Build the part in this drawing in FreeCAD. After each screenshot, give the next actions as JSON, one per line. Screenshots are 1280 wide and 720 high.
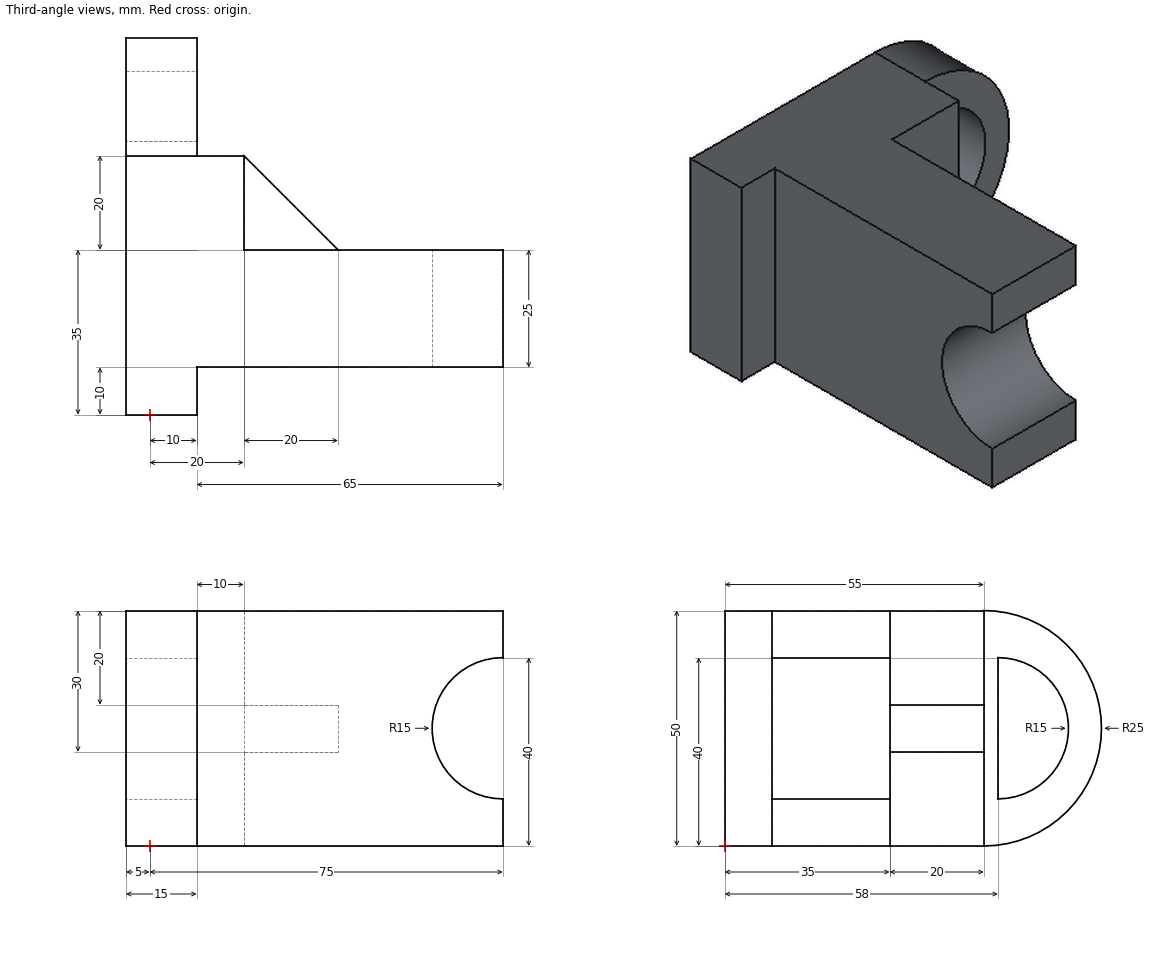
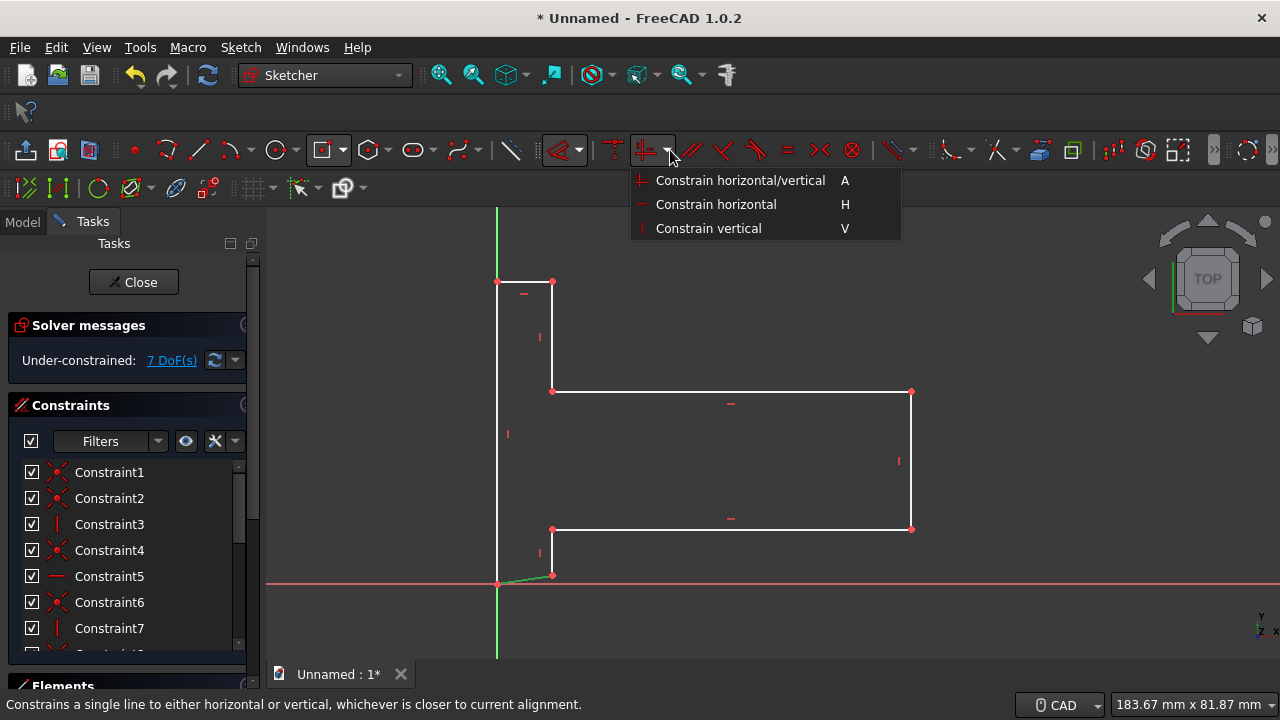
{"action": "left_click", "coordinate": [766, 204]}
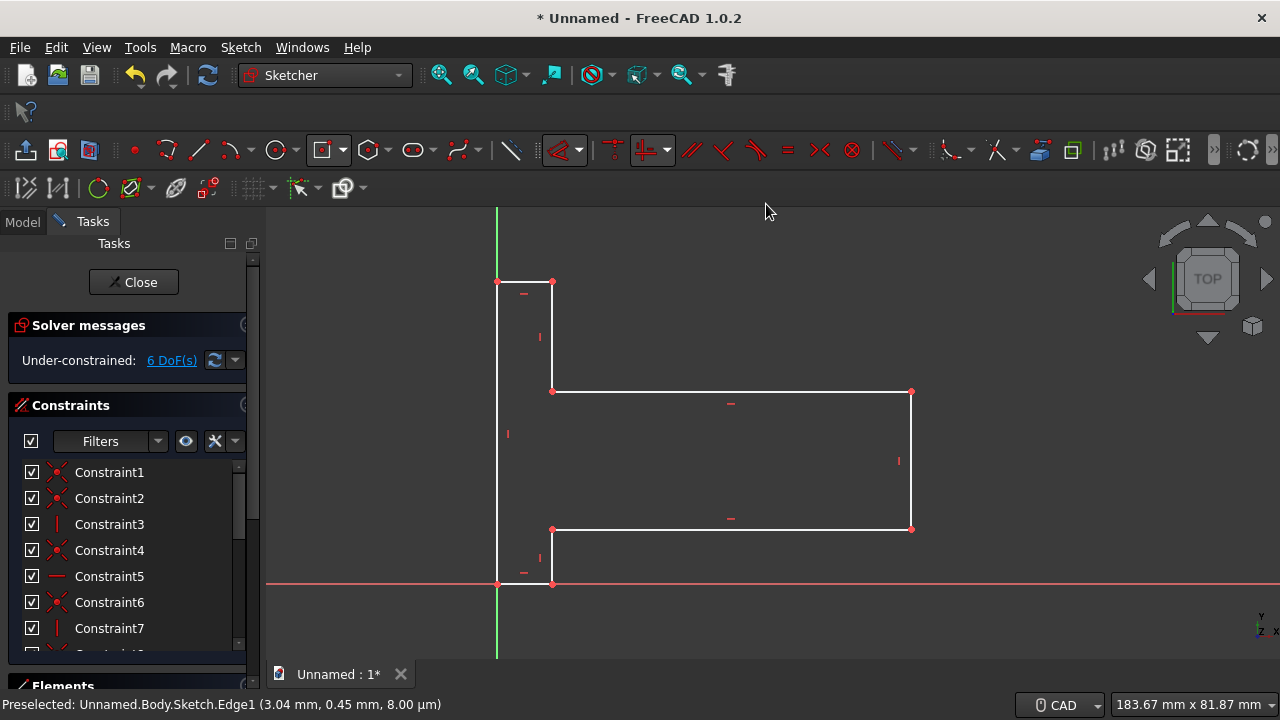
{"action": "left_click", "coordinate": [514, 584]}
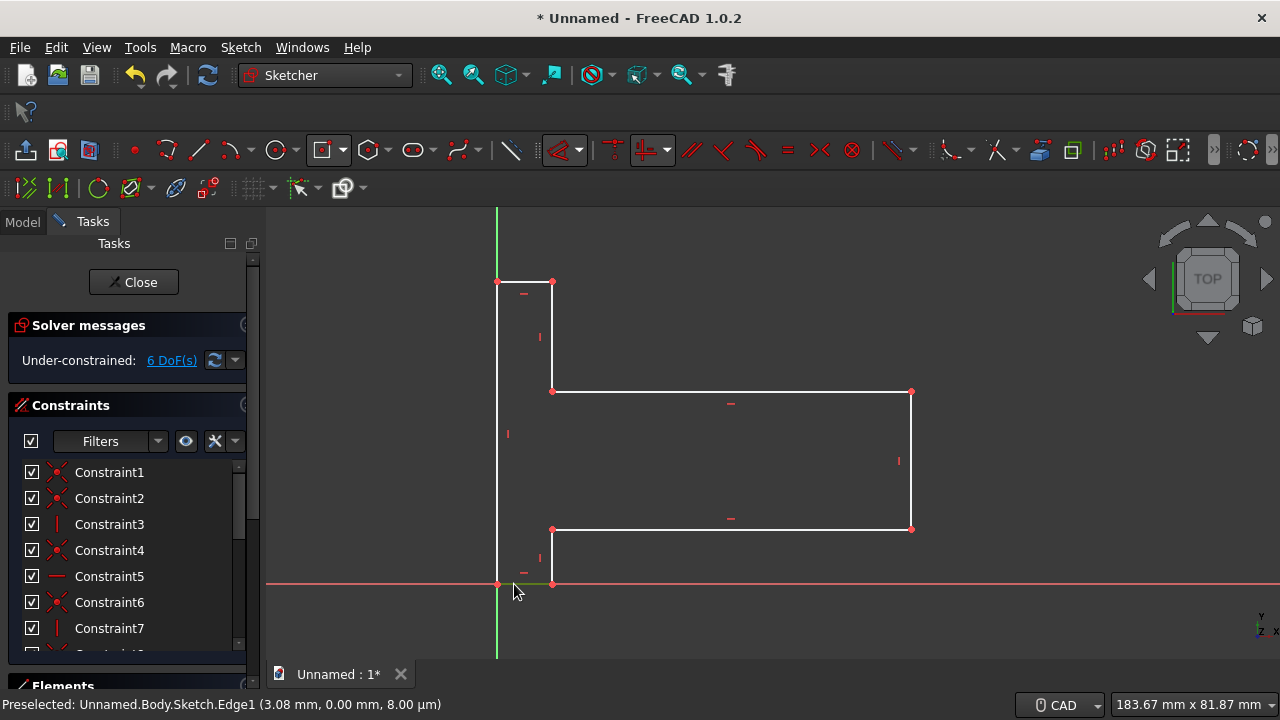
{"action": "left_click", "coordinate": [582, 150]}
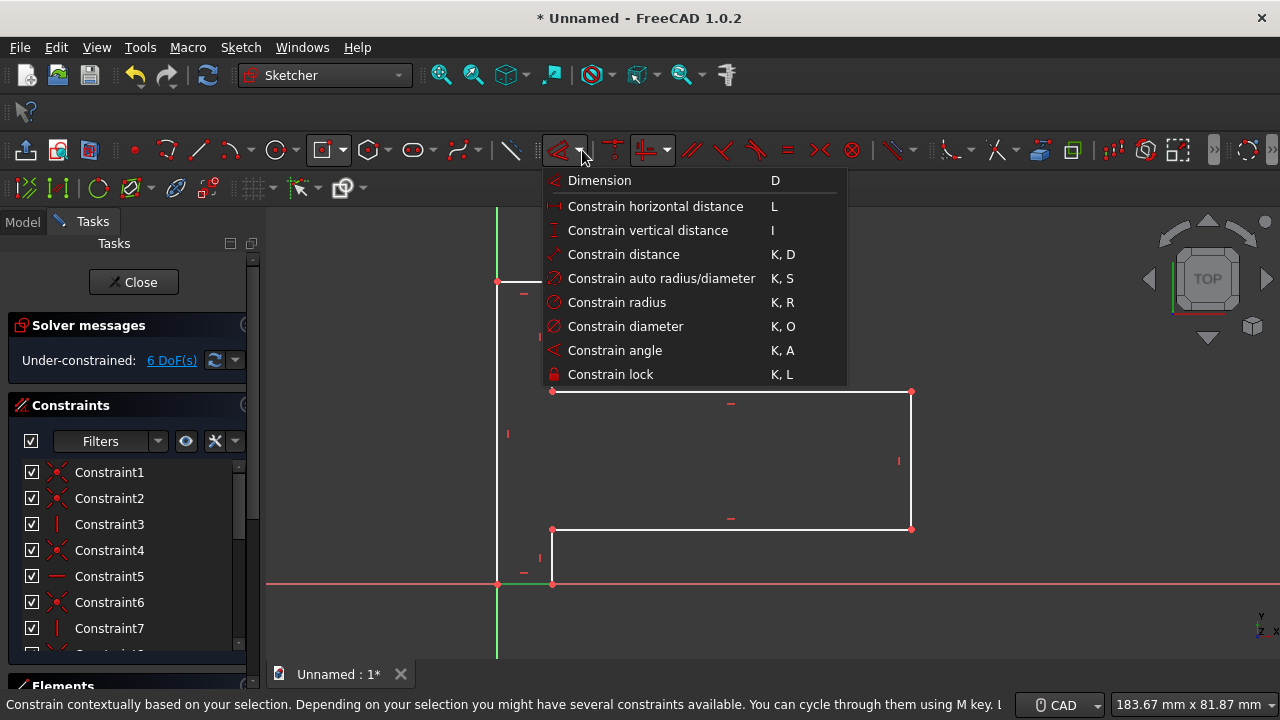
{"action": "left_click", "coordinate": [695, 206]}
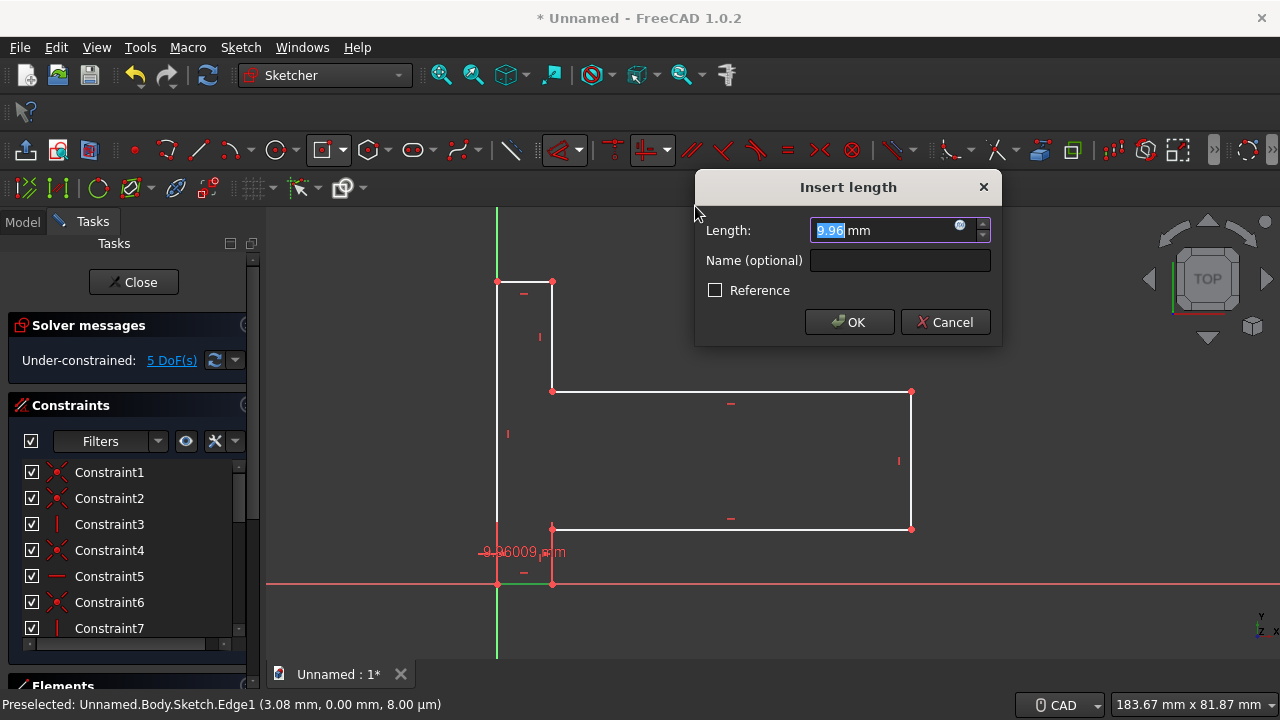
{"action": "type", "text": "10"}
{"action": "key", "text": "Return"}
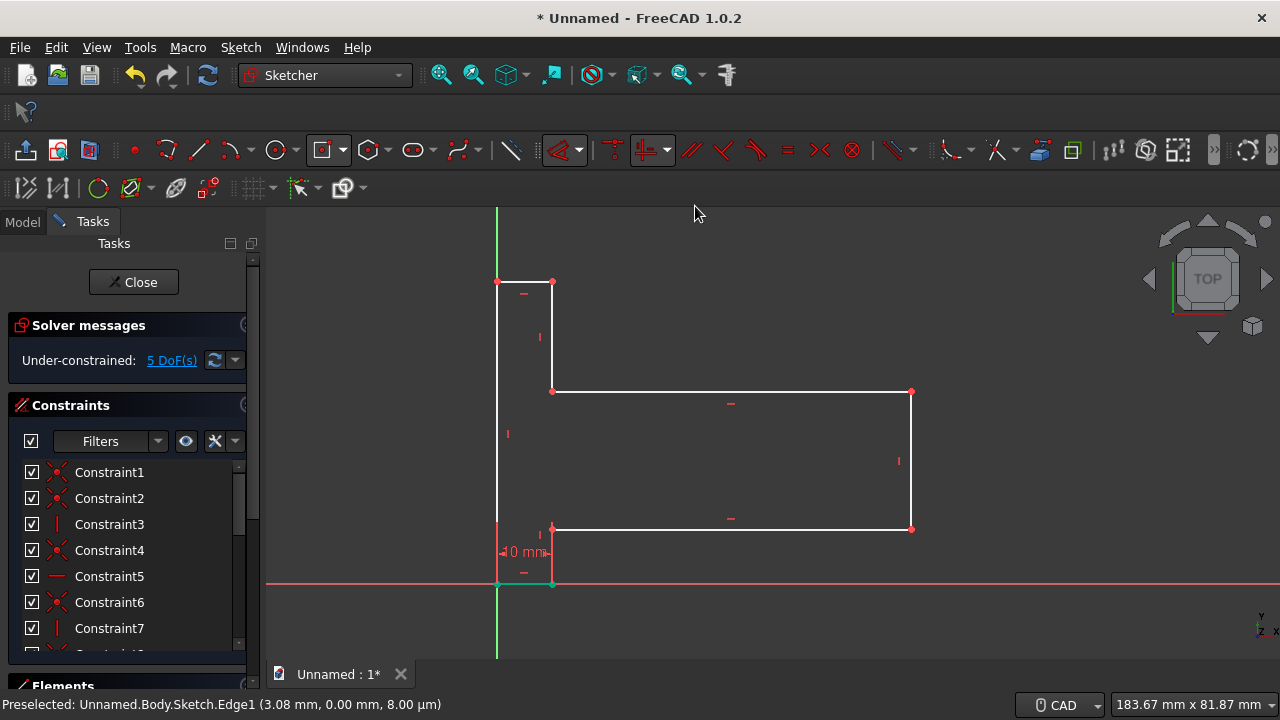
{"action": "left_click", "coordinate": [552, 568]}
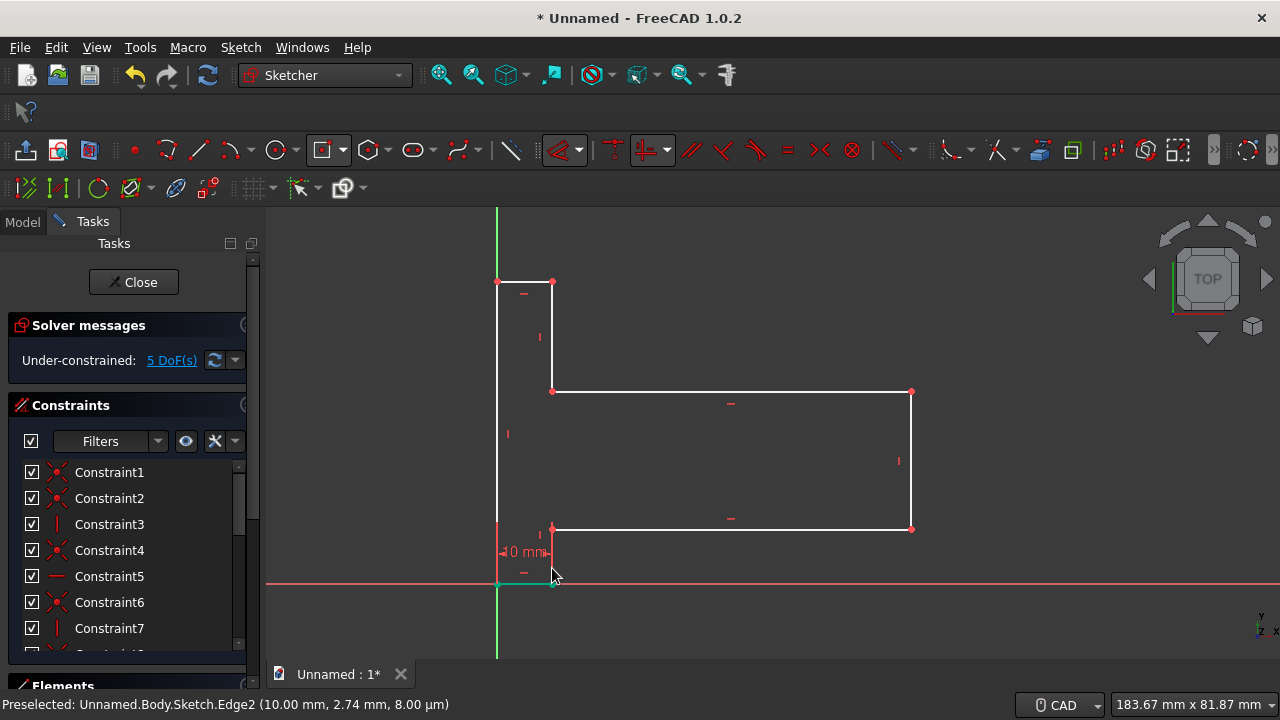
{"action": "key", "text": "i"}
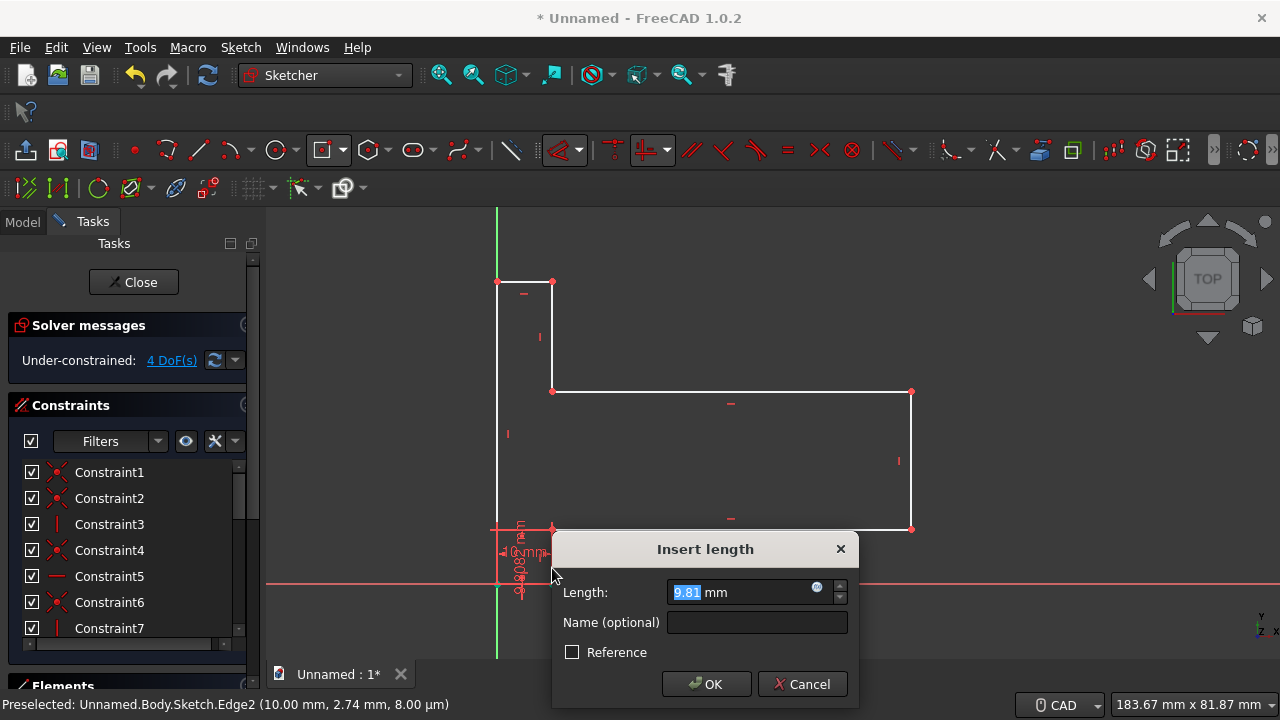
{"action": "type", "text": "10"}
{"action": "key", "text": "Return"}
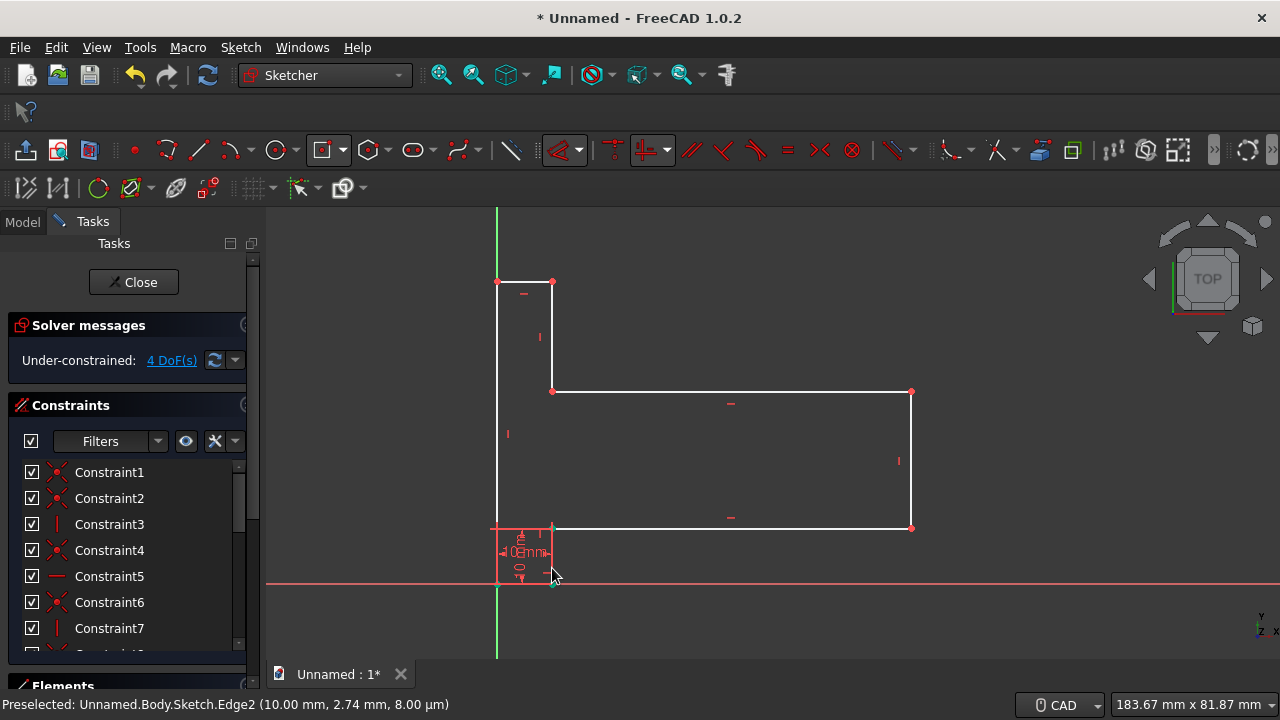
{"action": "left_click", "coordinate": [660, 529]}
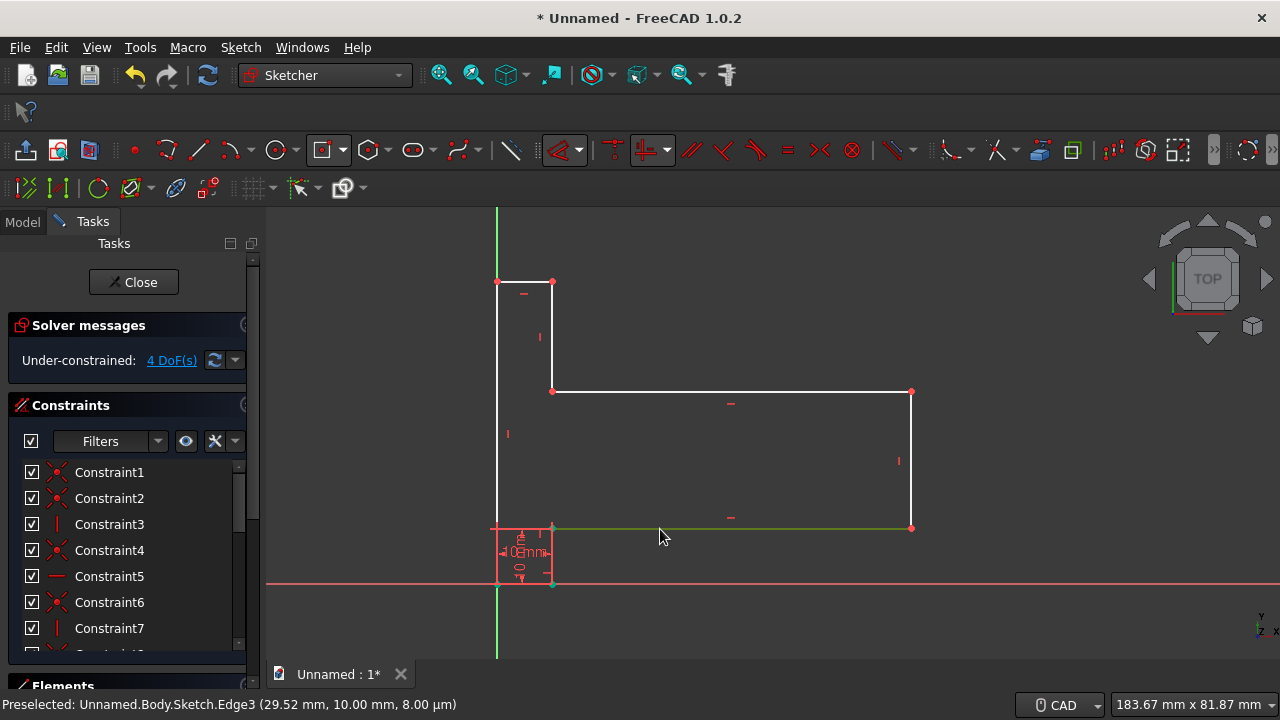
{"action": "key", "text": "l"}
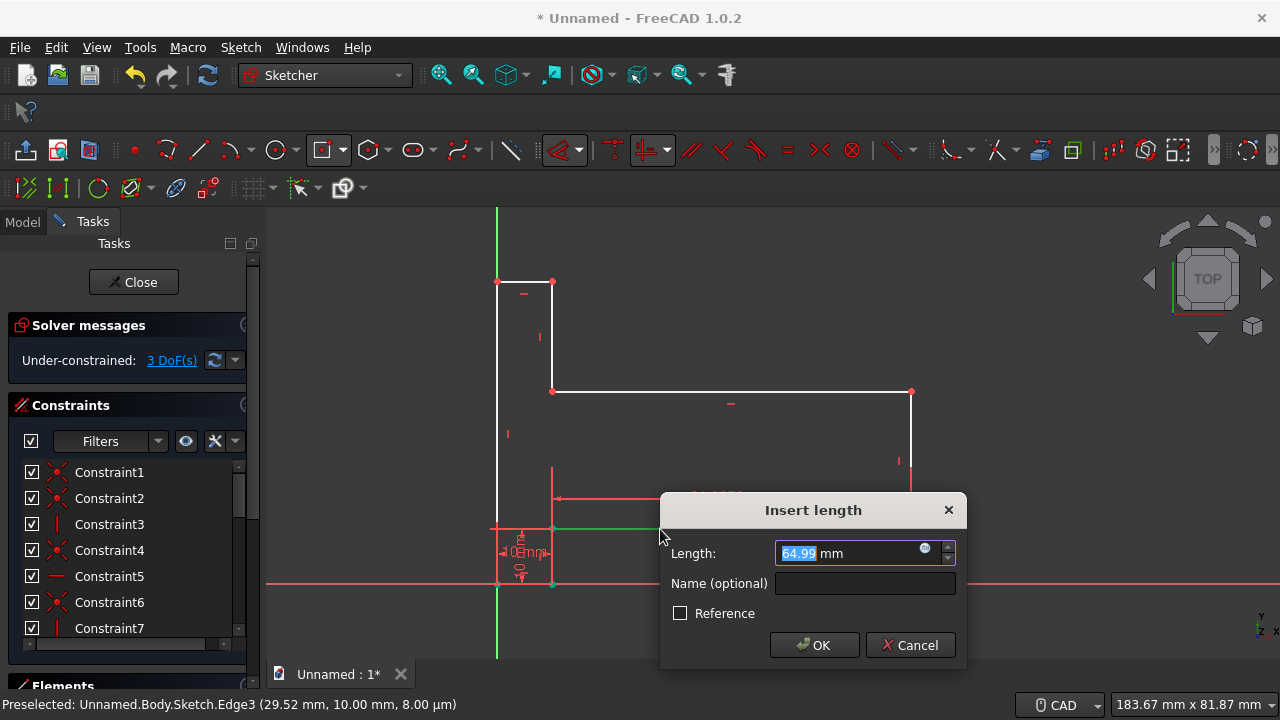
{"action": "type", "text": "65"}
{"action": "key", "text": "Return"}